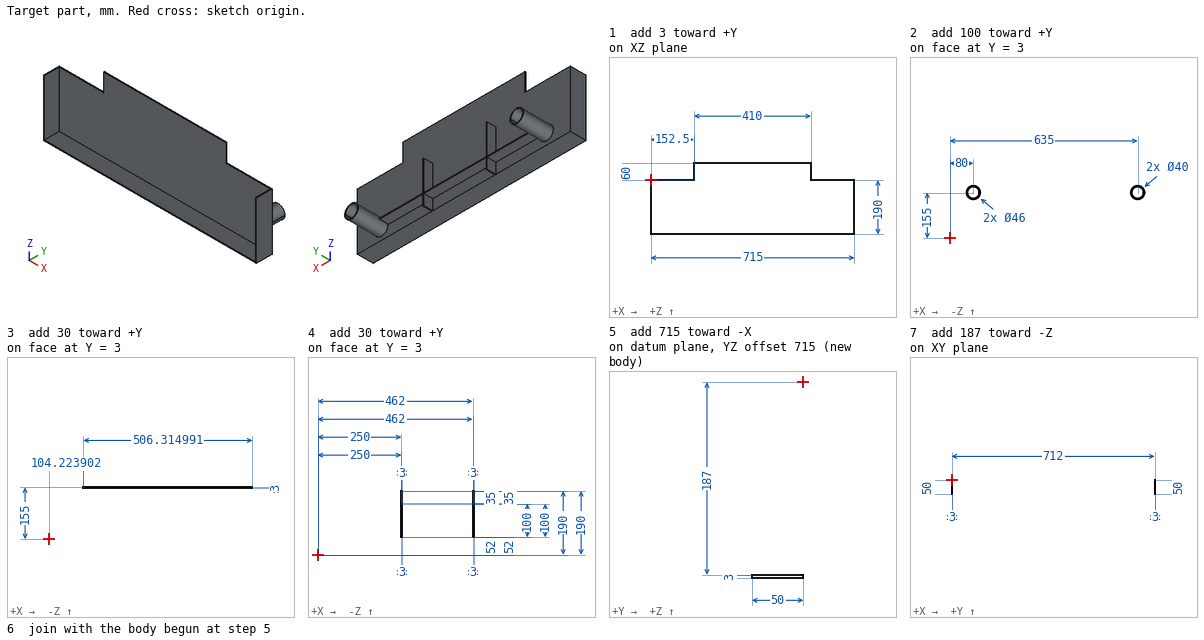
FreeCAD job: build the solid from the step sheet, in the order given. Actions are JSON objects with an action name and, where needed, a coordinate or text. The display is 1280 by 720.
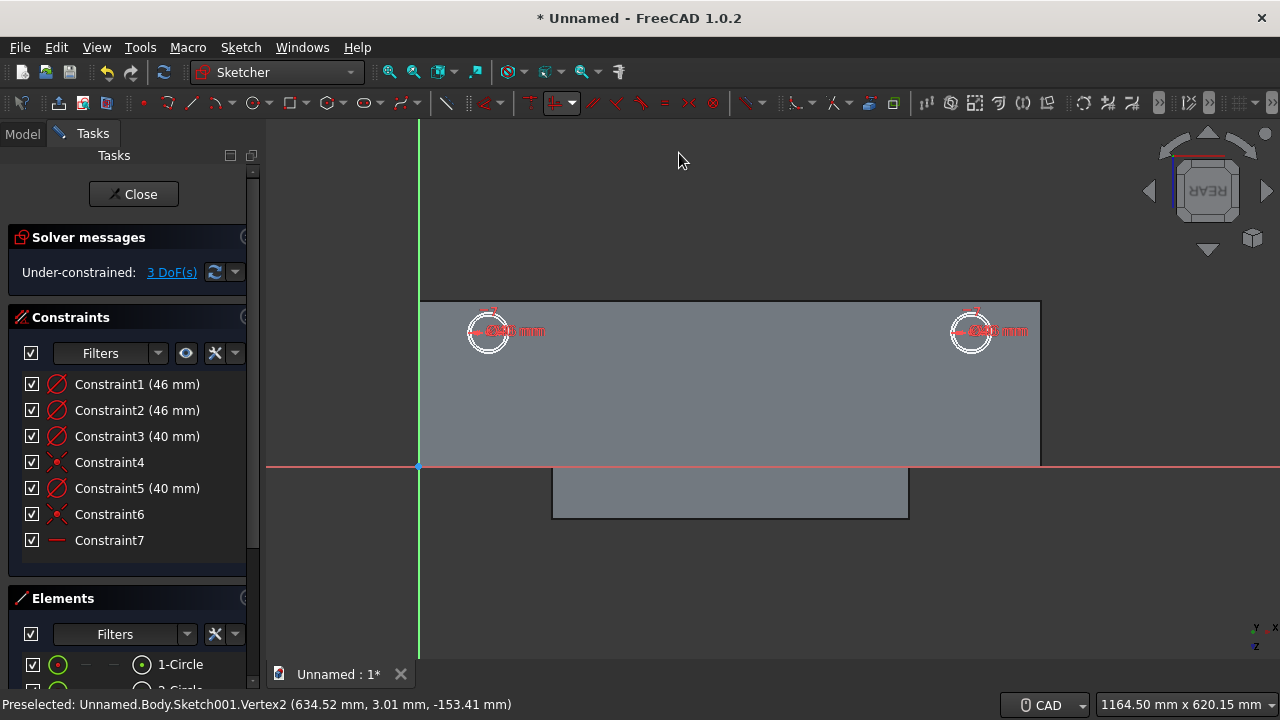
{"action": "key", "text": "d"}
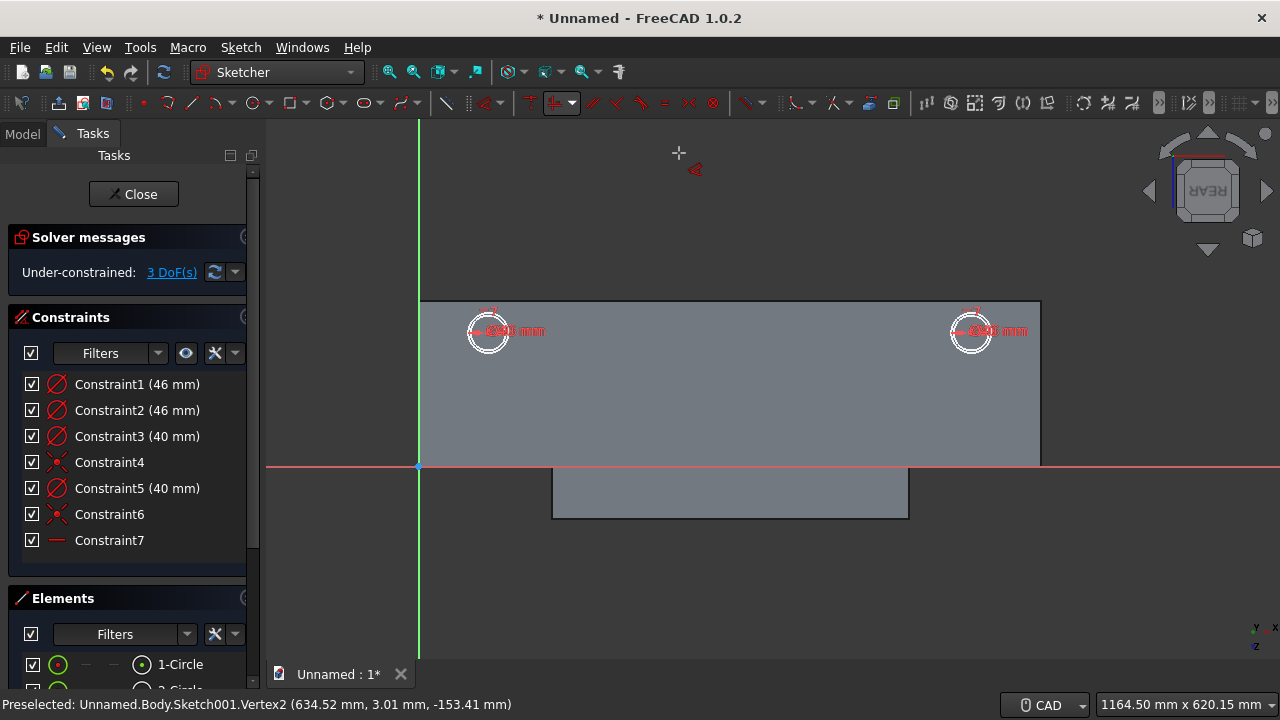
{"action": "left_click", "coordinate": [488, 333]}
{"action": "left_click", "coordinate": [454, 501]}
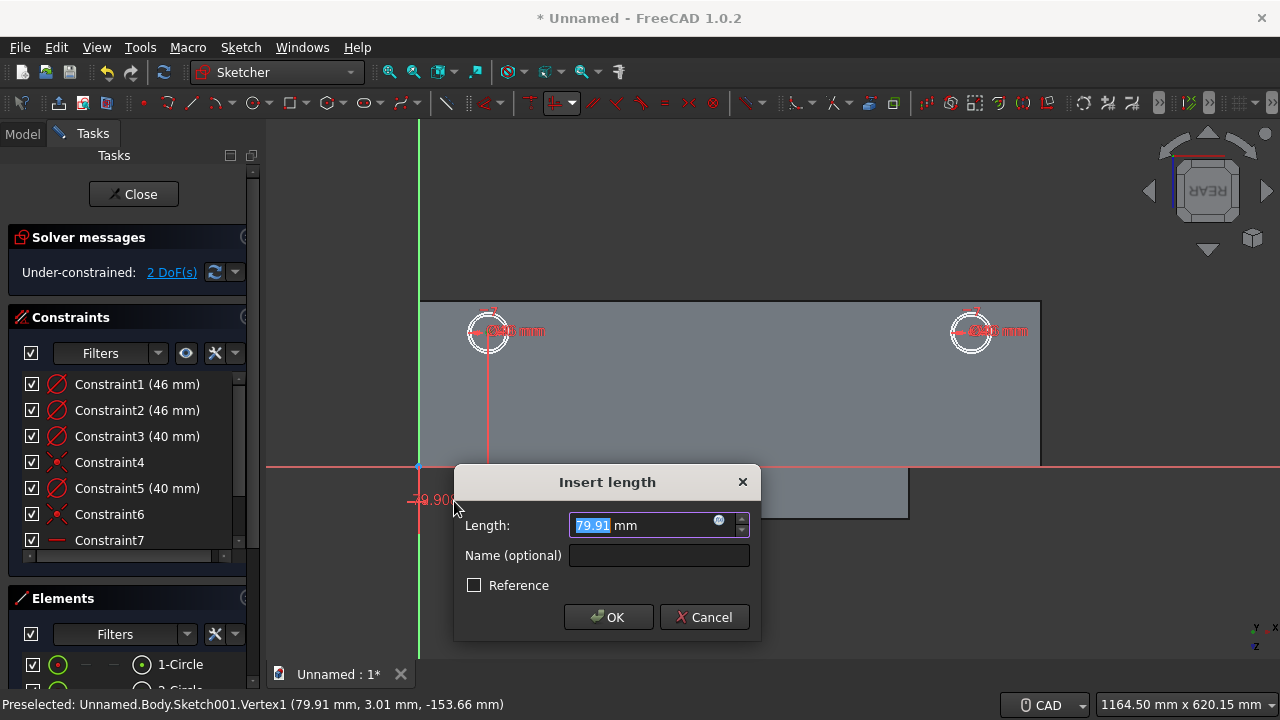
{"action": "type", "text": "80"}
{"action": "key", "text": "Return"}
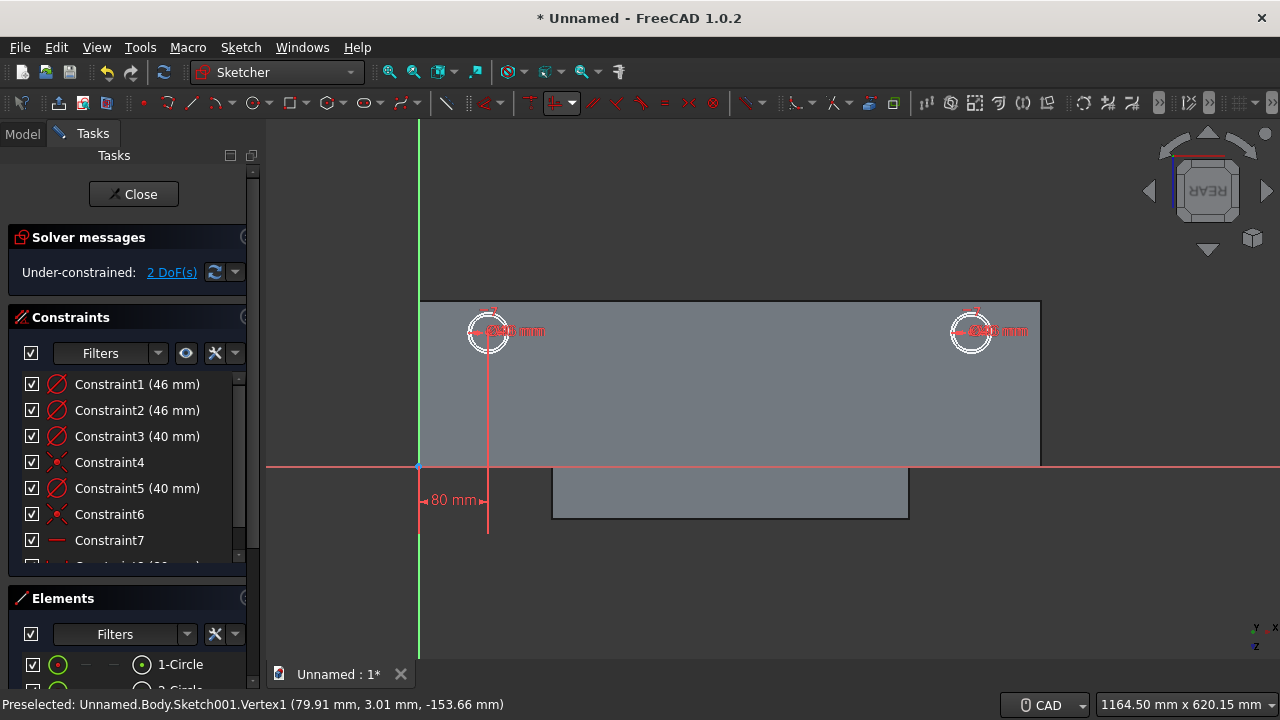
{"action": "left_click", "coordinate": [488, 333]}
{"action": "left_click", "coordinate": [385, 400]}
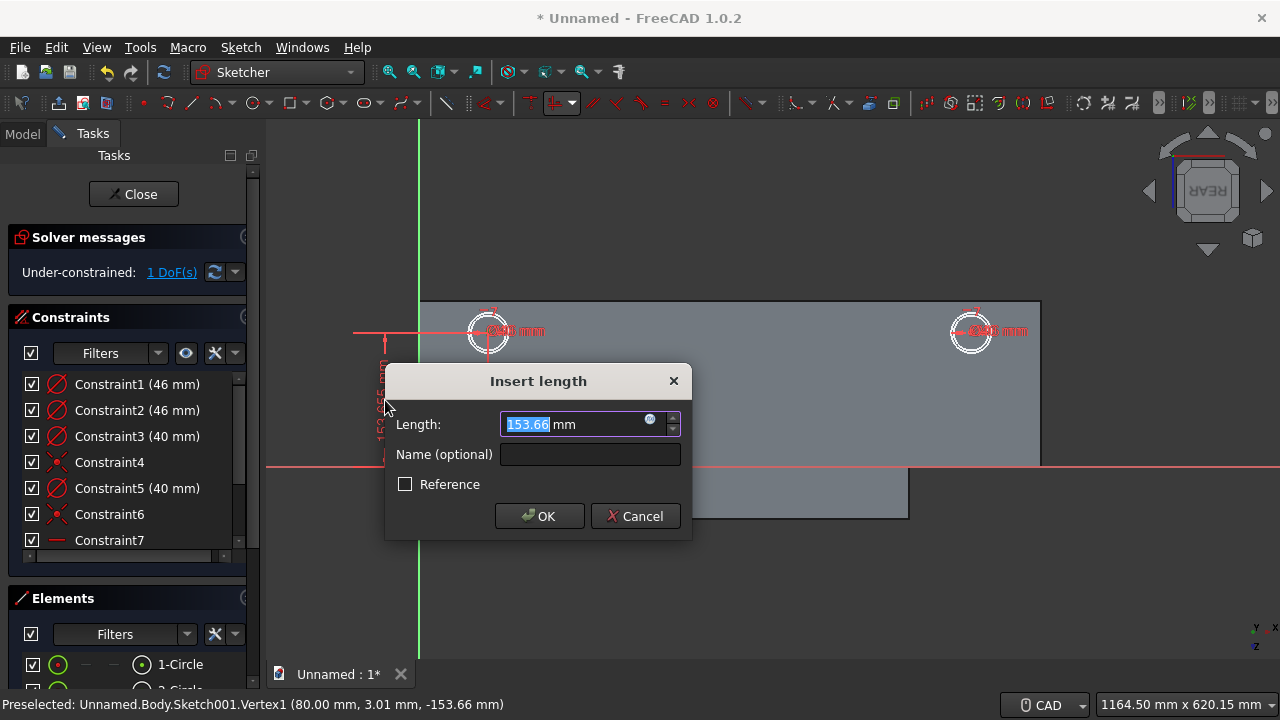
{"action": "type", "text": "155"}
{"action": "key", "text": "Return"}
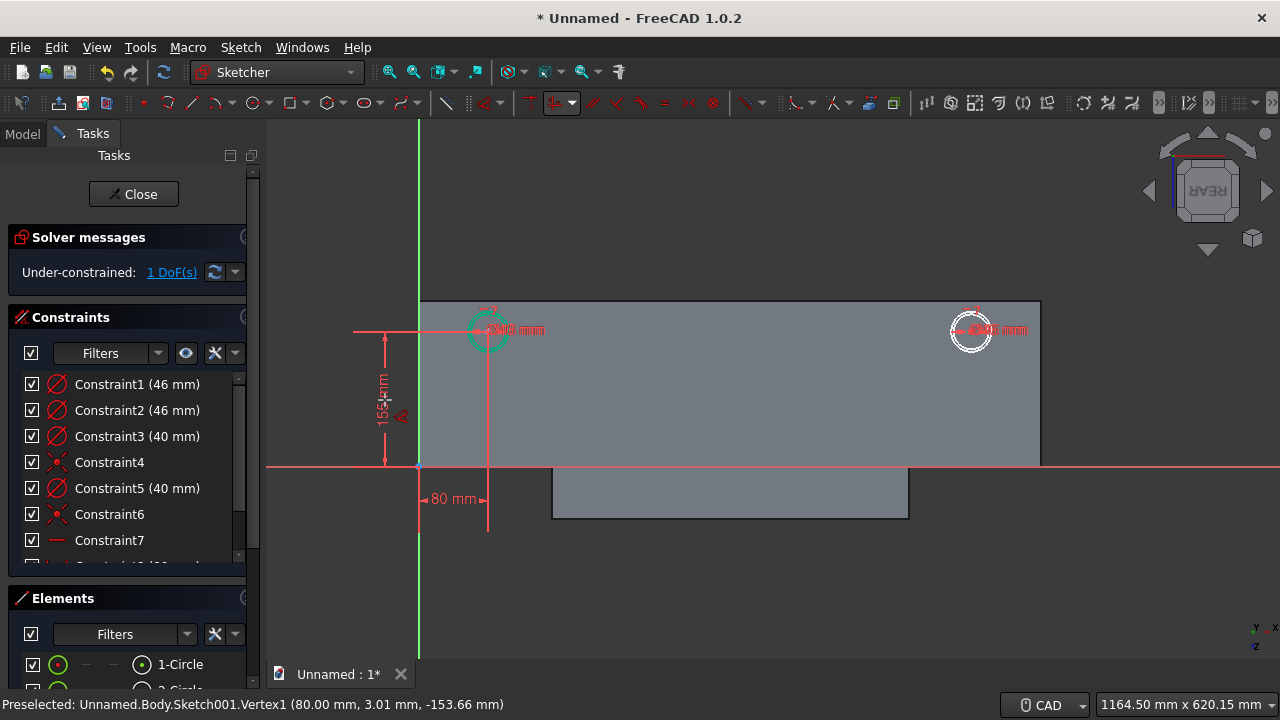
{"action": "left_click", "coordinate": [971, 332]}
{"action": "left_click", "coordinate": [695, 501]}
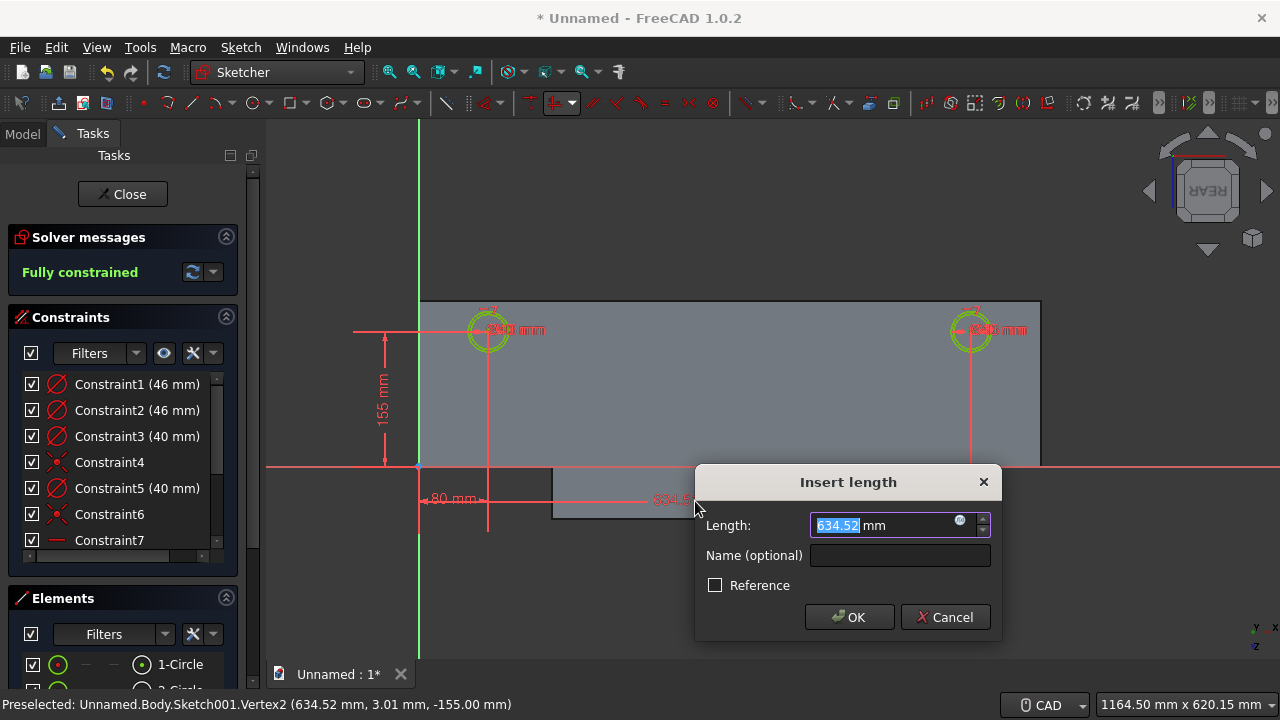
{"action": "type", "text": "635"}
{"action": "key", "text": "Return"}
{"action": "key", "text": "Escape"}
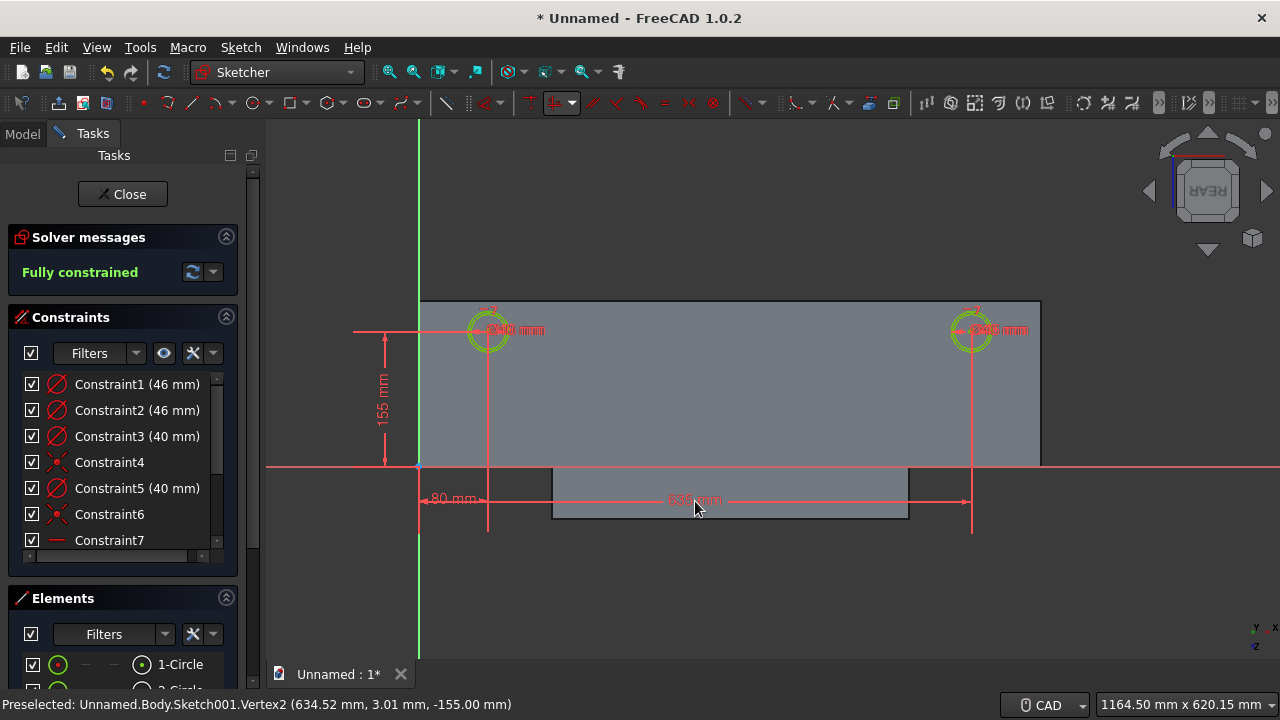
{"action": "left_click", "coordinate": [123, 194]}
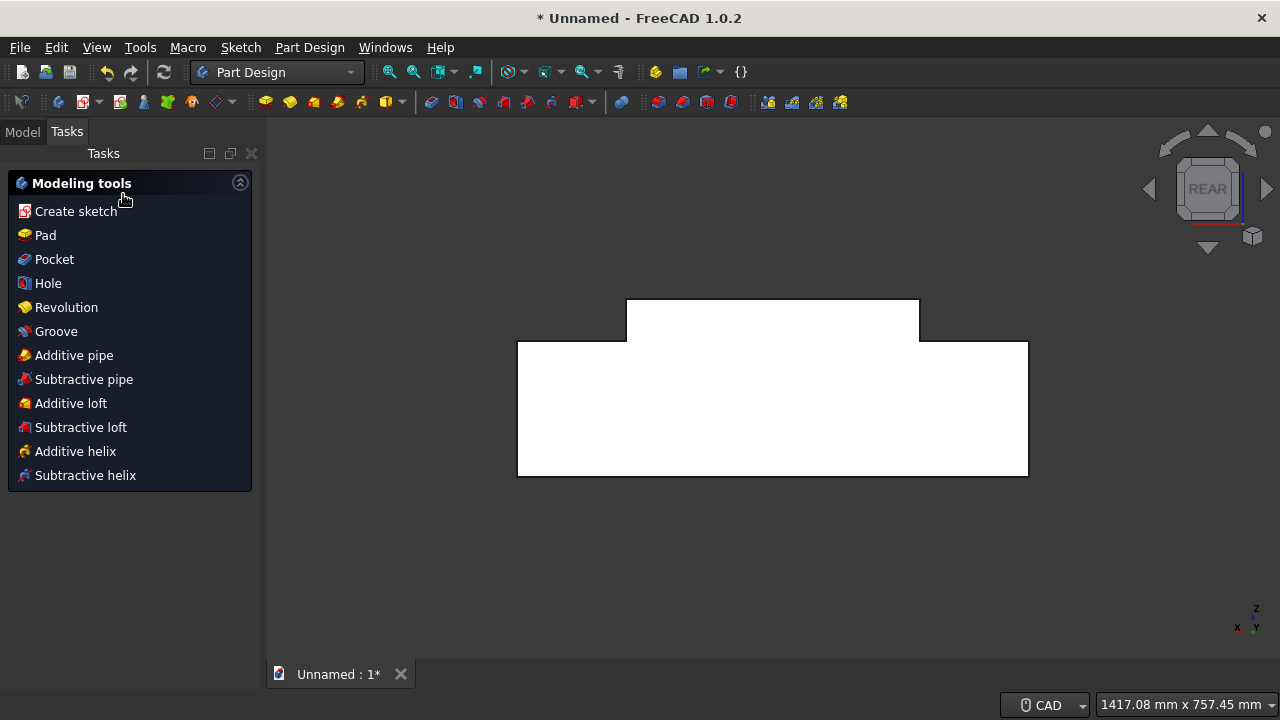
{"action": "left_click", "coordinate": [266, 102]}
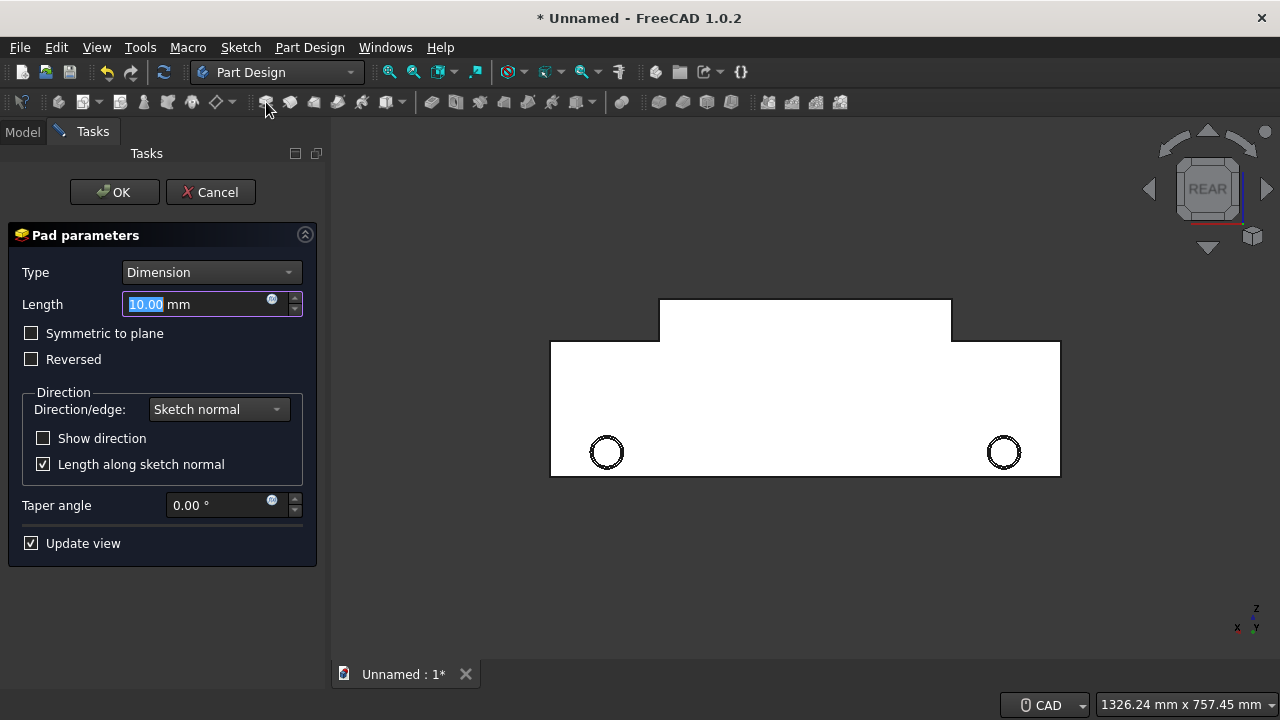
{"action": "type", "text": "100"}
{"action": "key", "text": "Tab"}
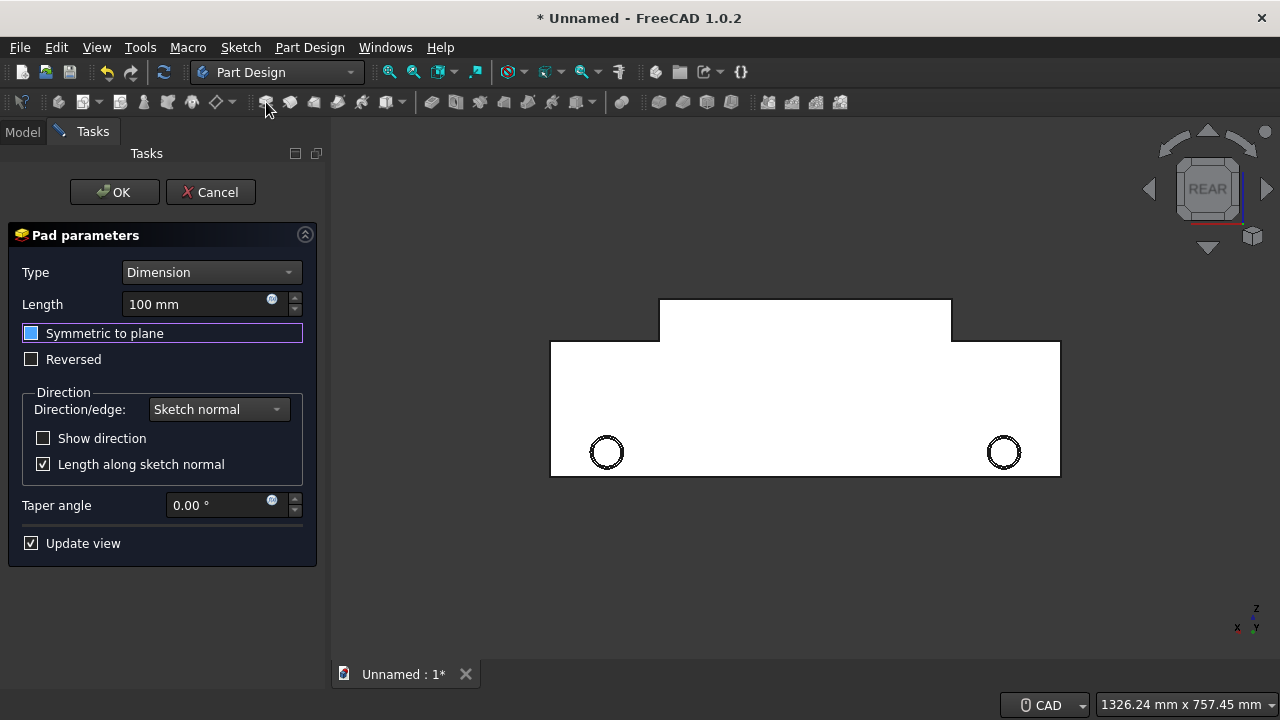
{"action": "left_click", "coordinate": [115, 192]}